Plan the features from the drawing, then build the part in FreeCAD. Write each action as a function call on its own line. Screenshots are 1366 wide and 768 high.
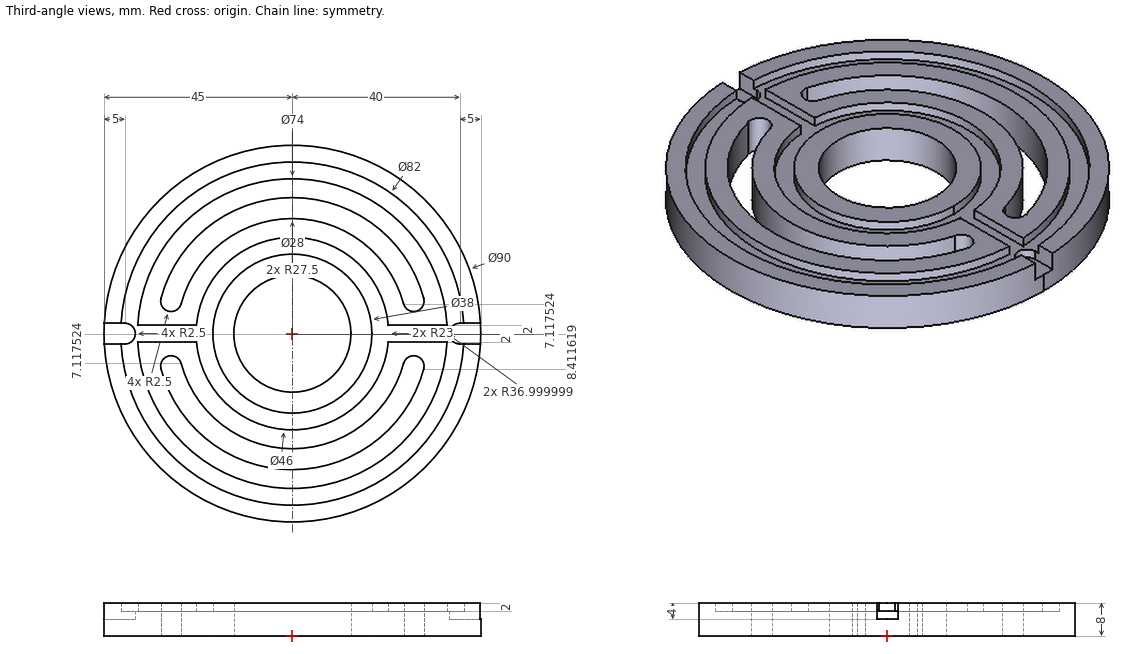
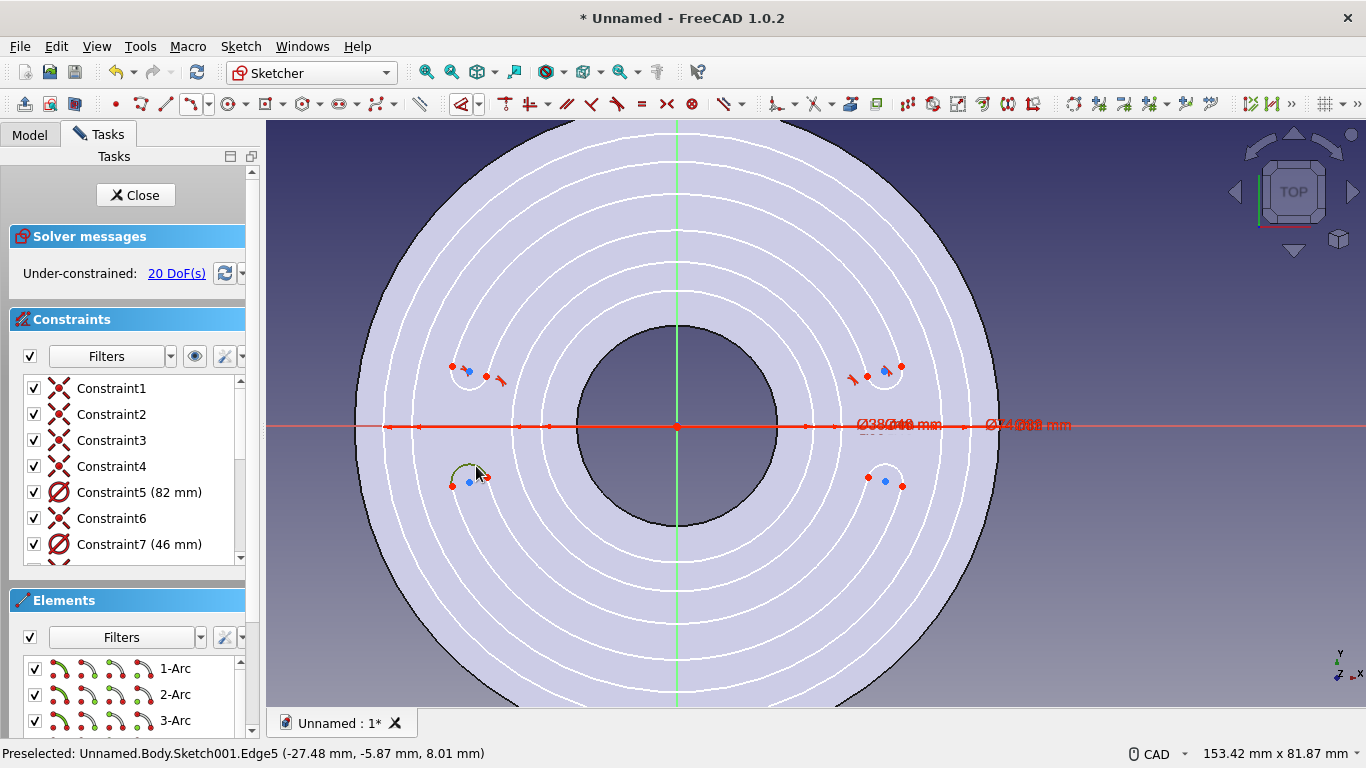
click(560, 629)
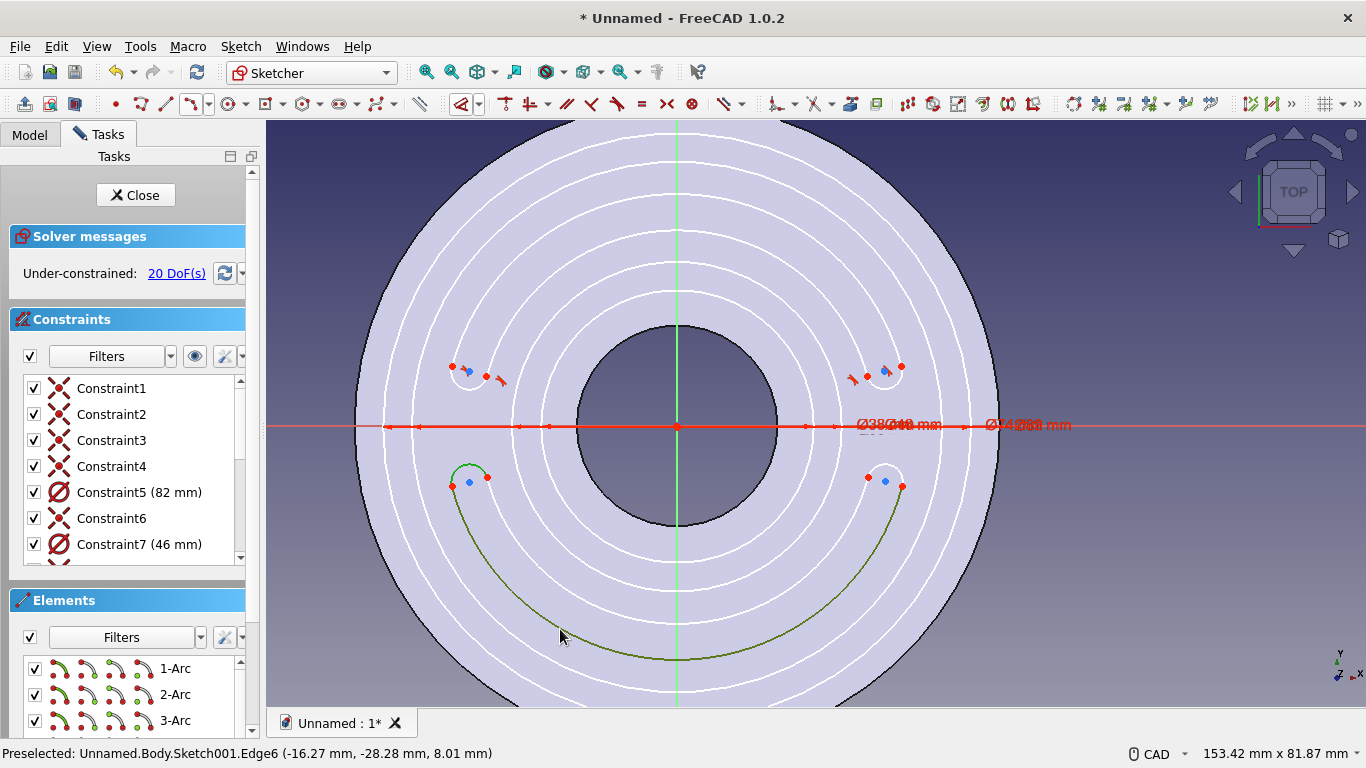
key(t)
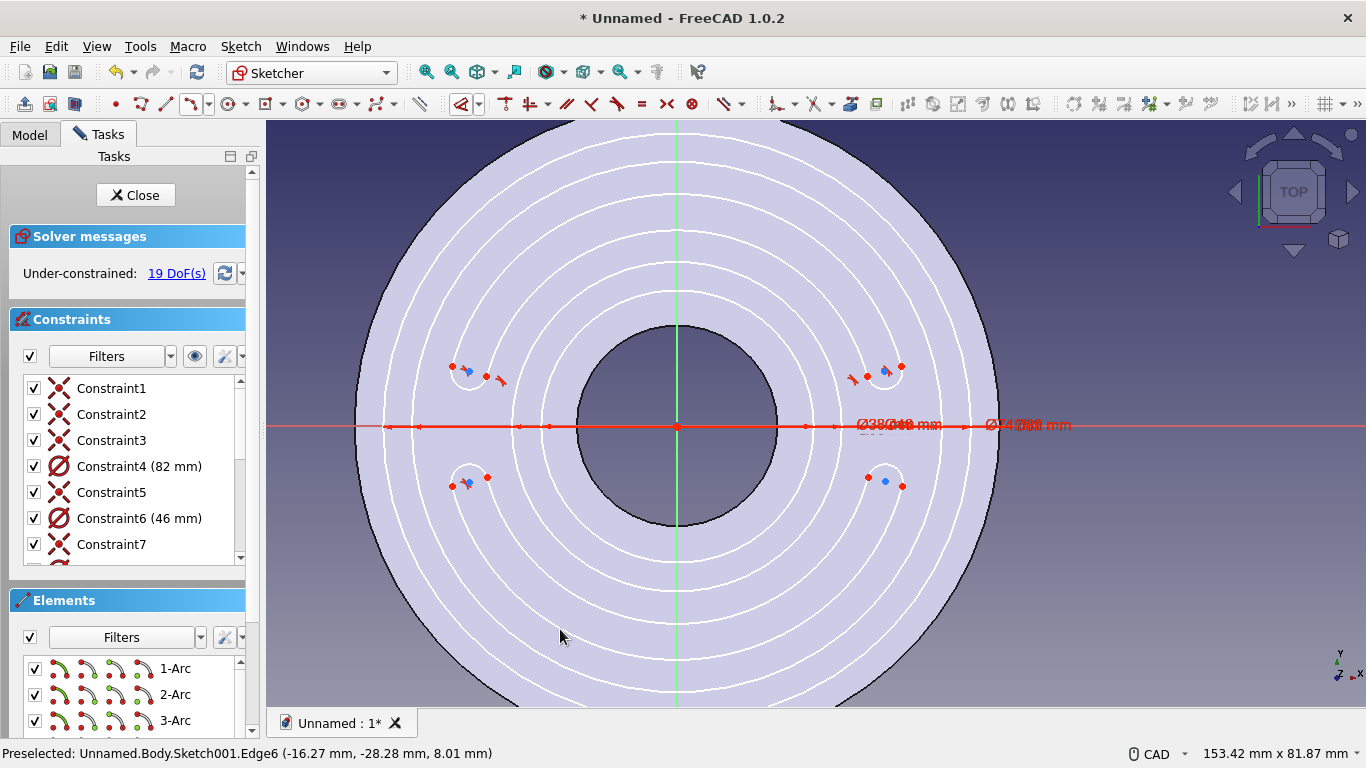
click(476, 466)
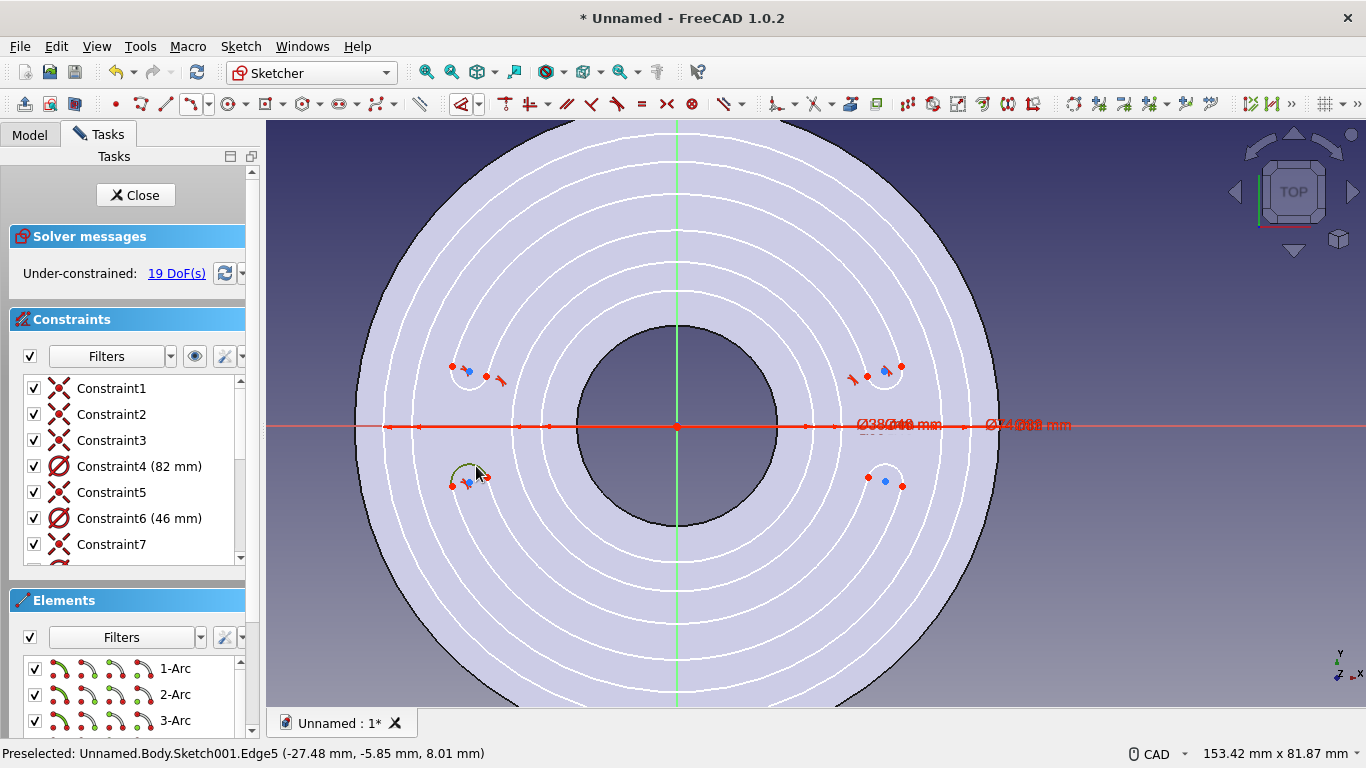
click(579, 597)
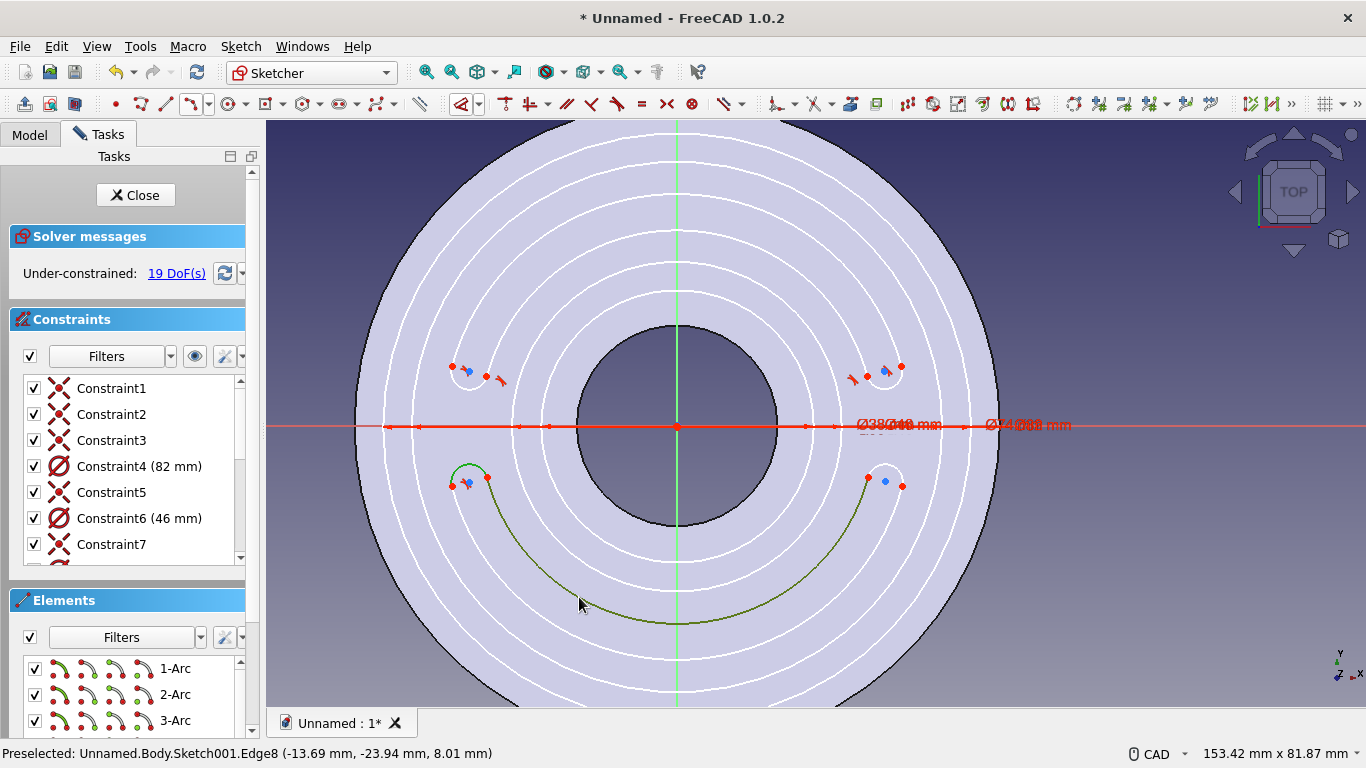
click(617, 104)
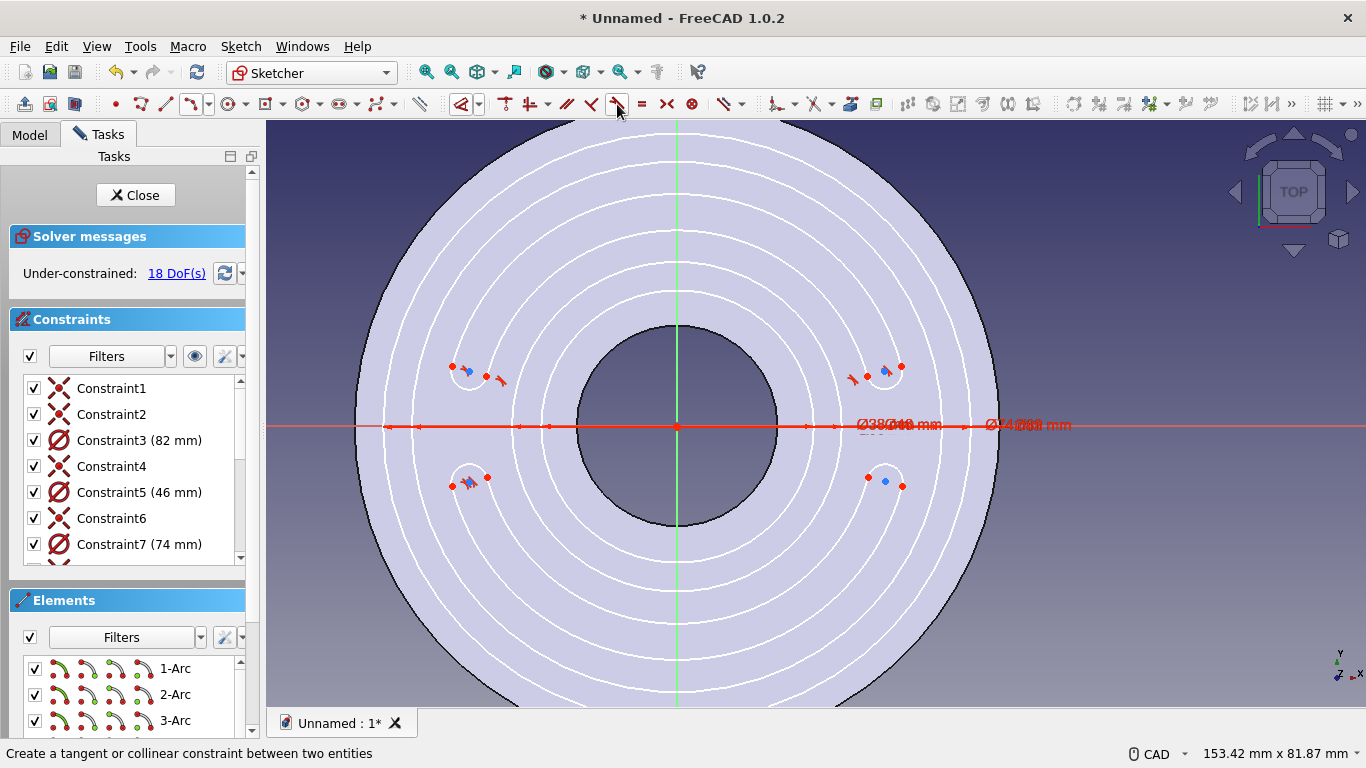
click(560, 629)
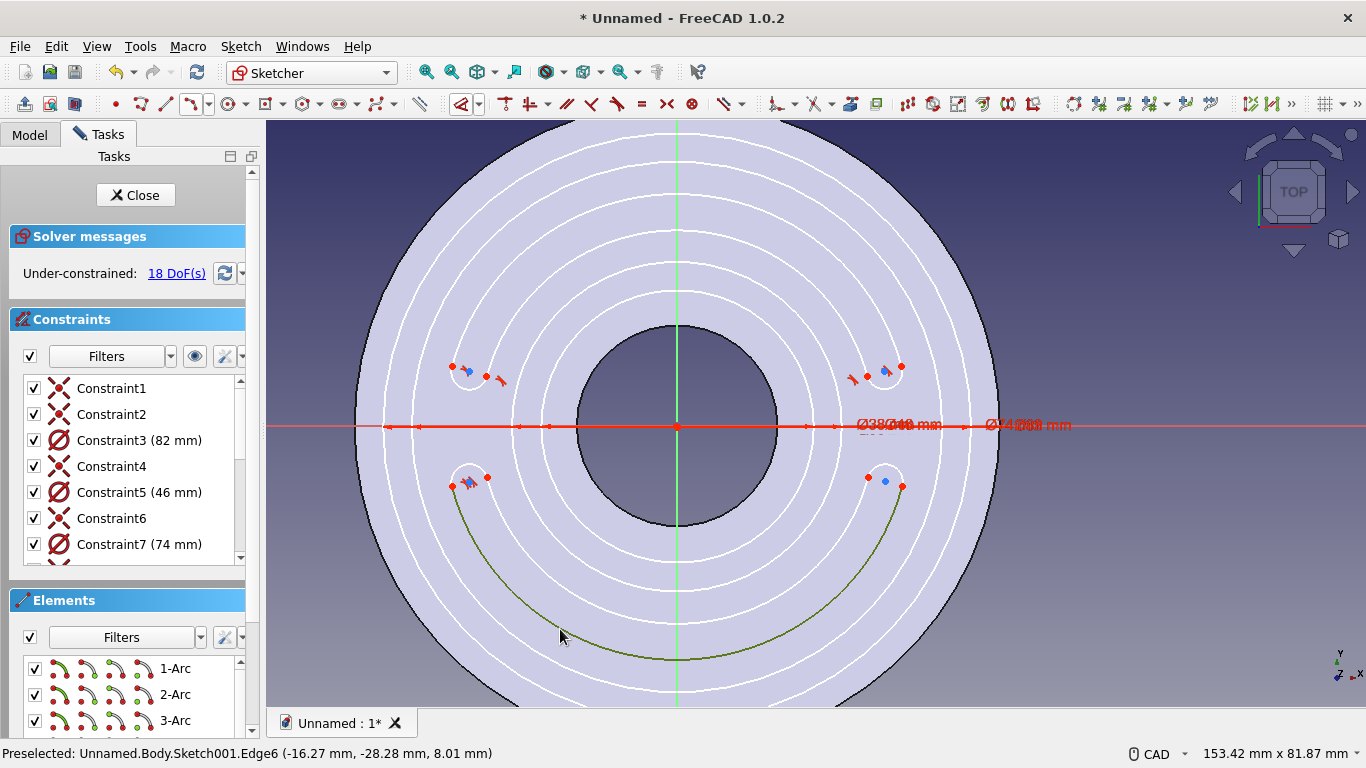
click(899, 471)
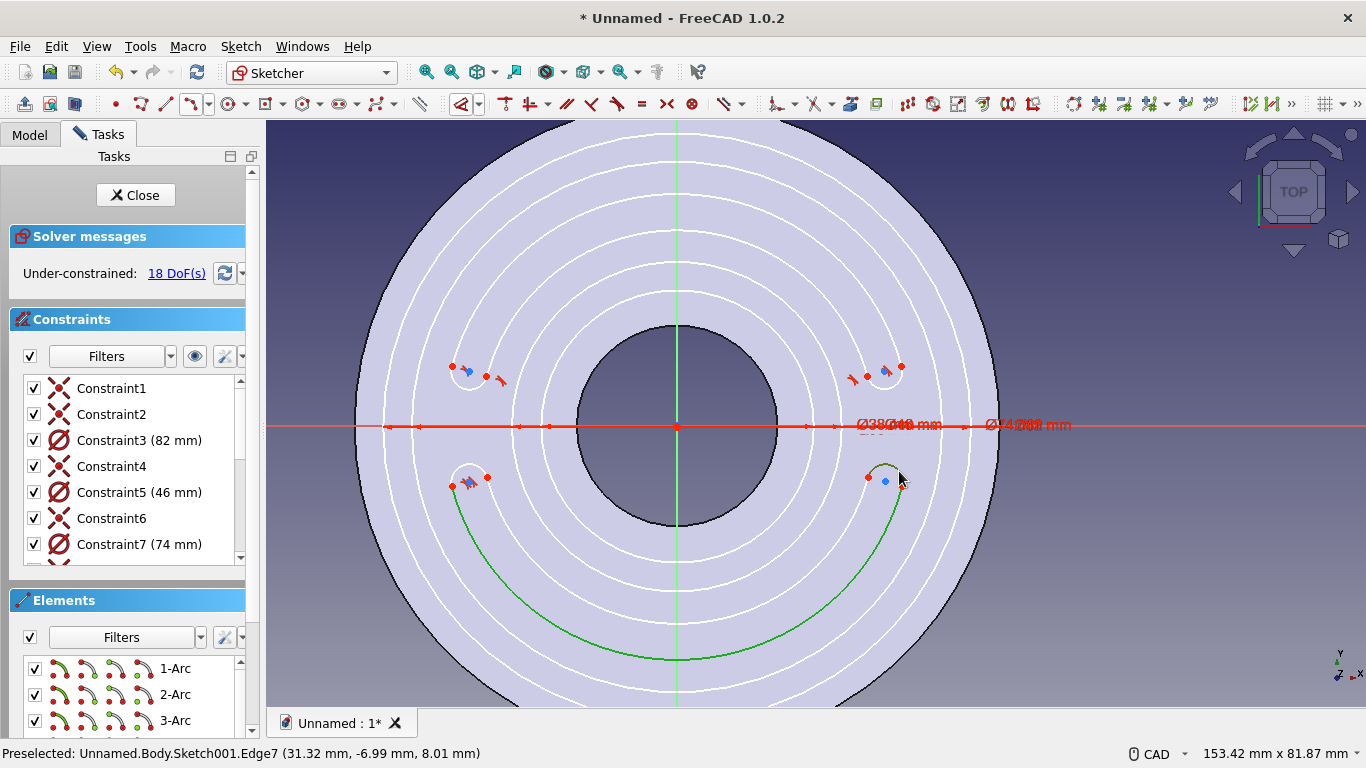
key(t)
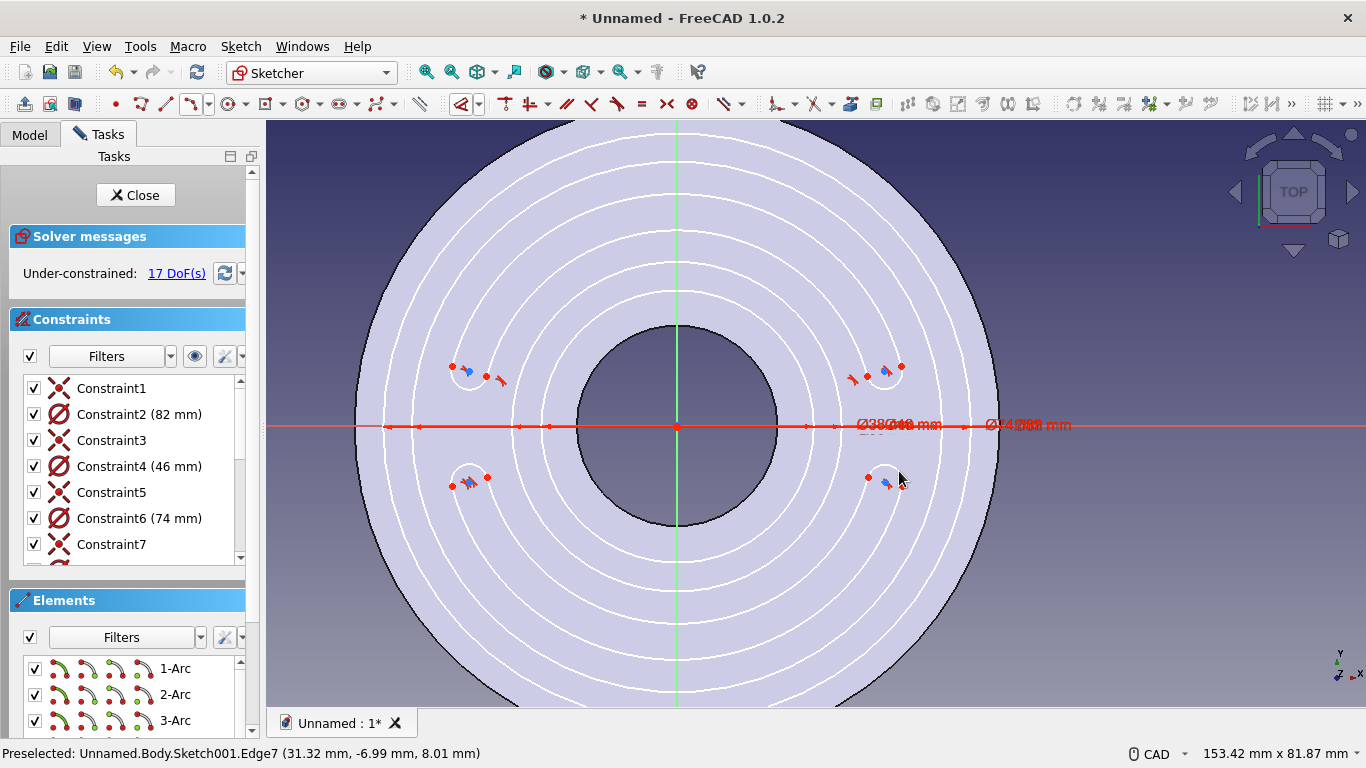
click(899, 471)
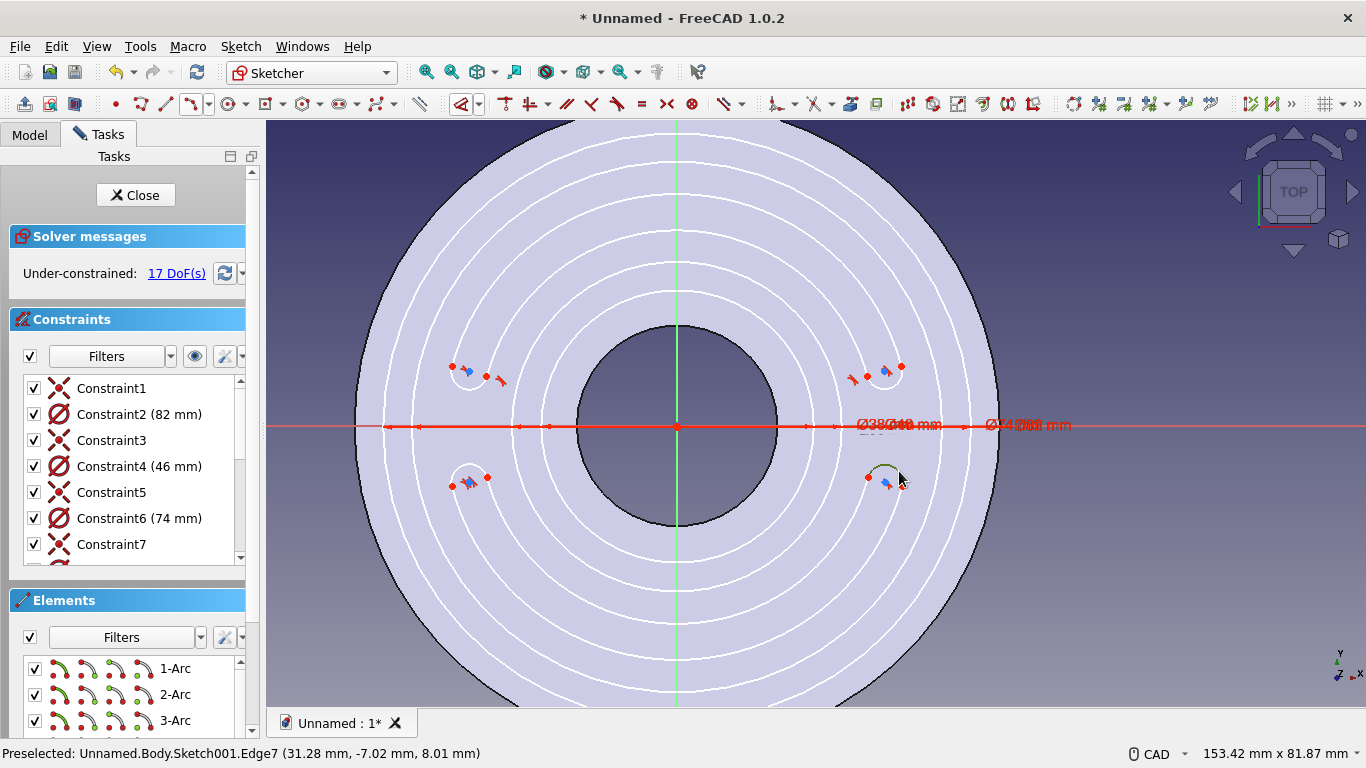
click(579, 597)